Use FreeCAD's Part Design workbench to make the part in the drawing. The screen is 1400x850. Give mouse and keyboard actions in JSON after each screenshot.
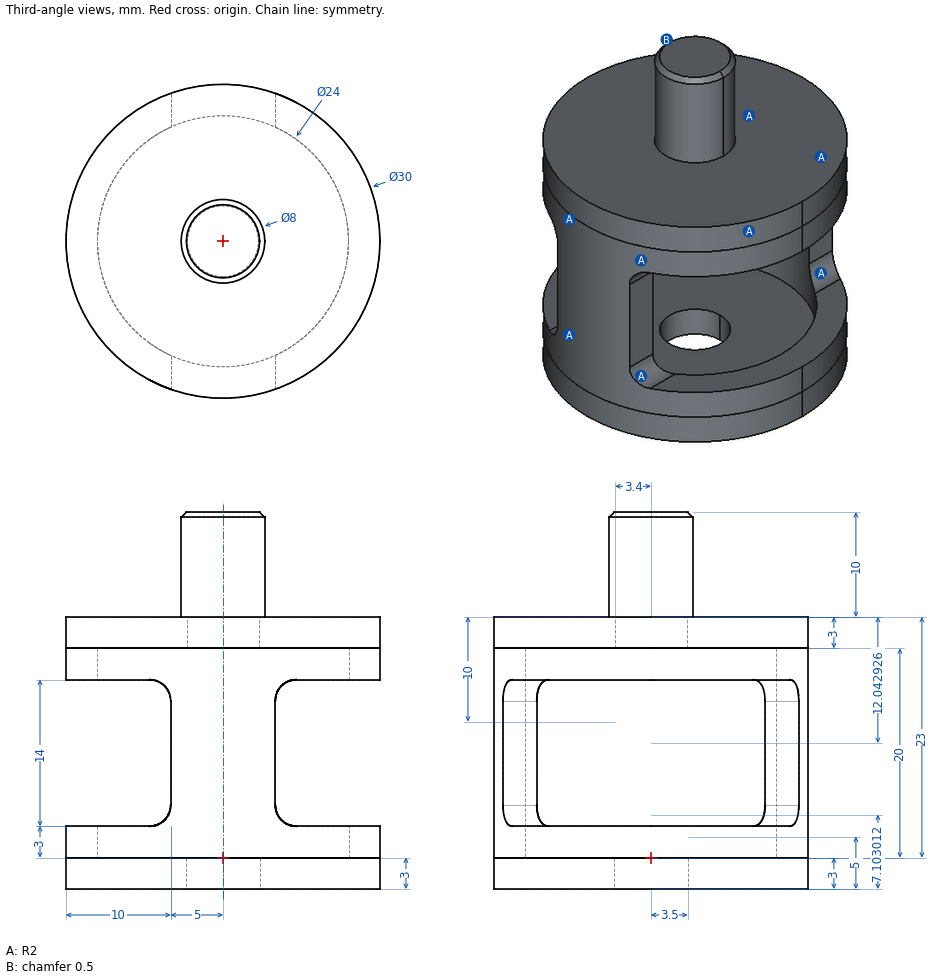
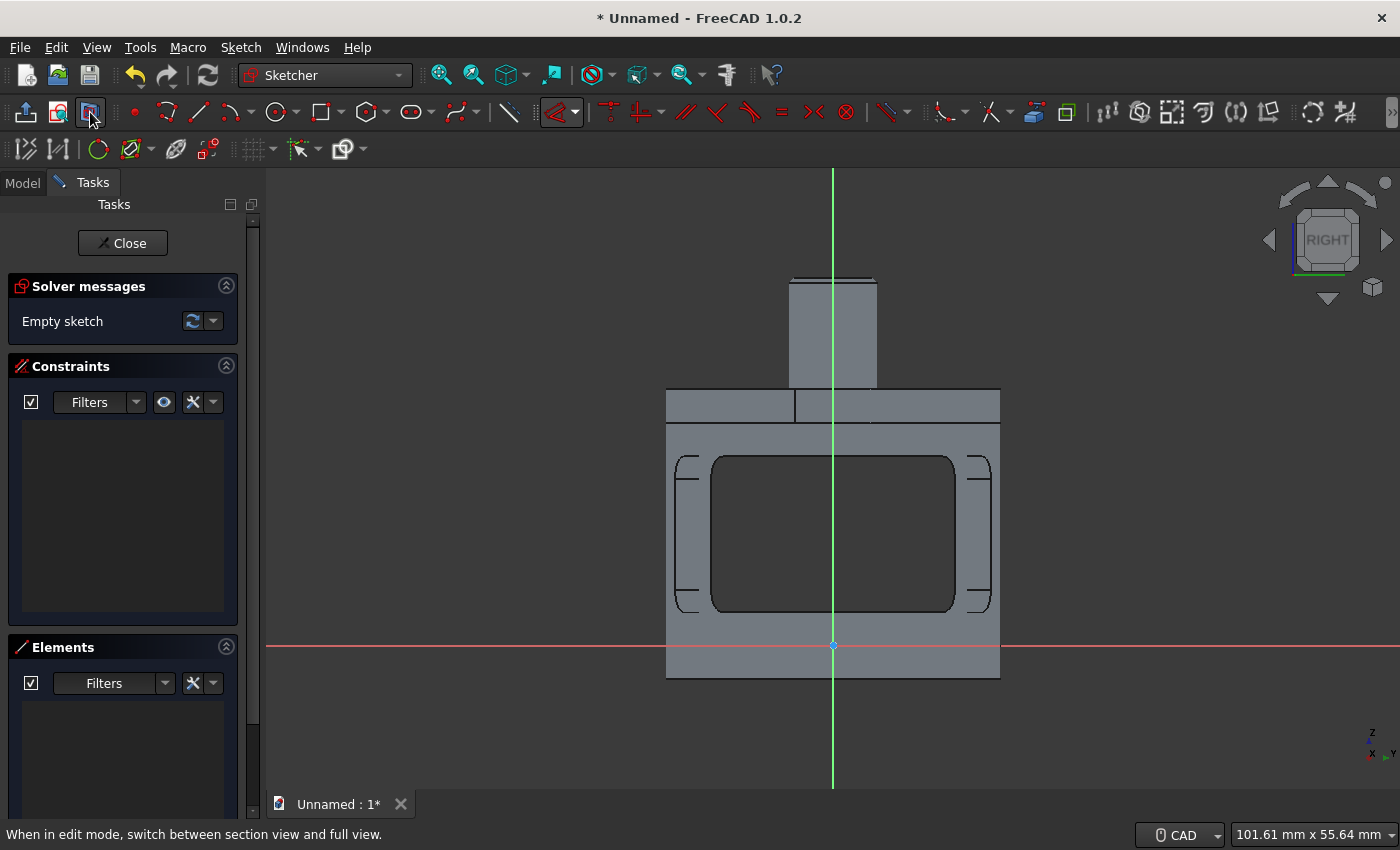
{"action": "scroll", "coordinate": [875, 681], "scroll_direction": "up", "scroll_amount": 8}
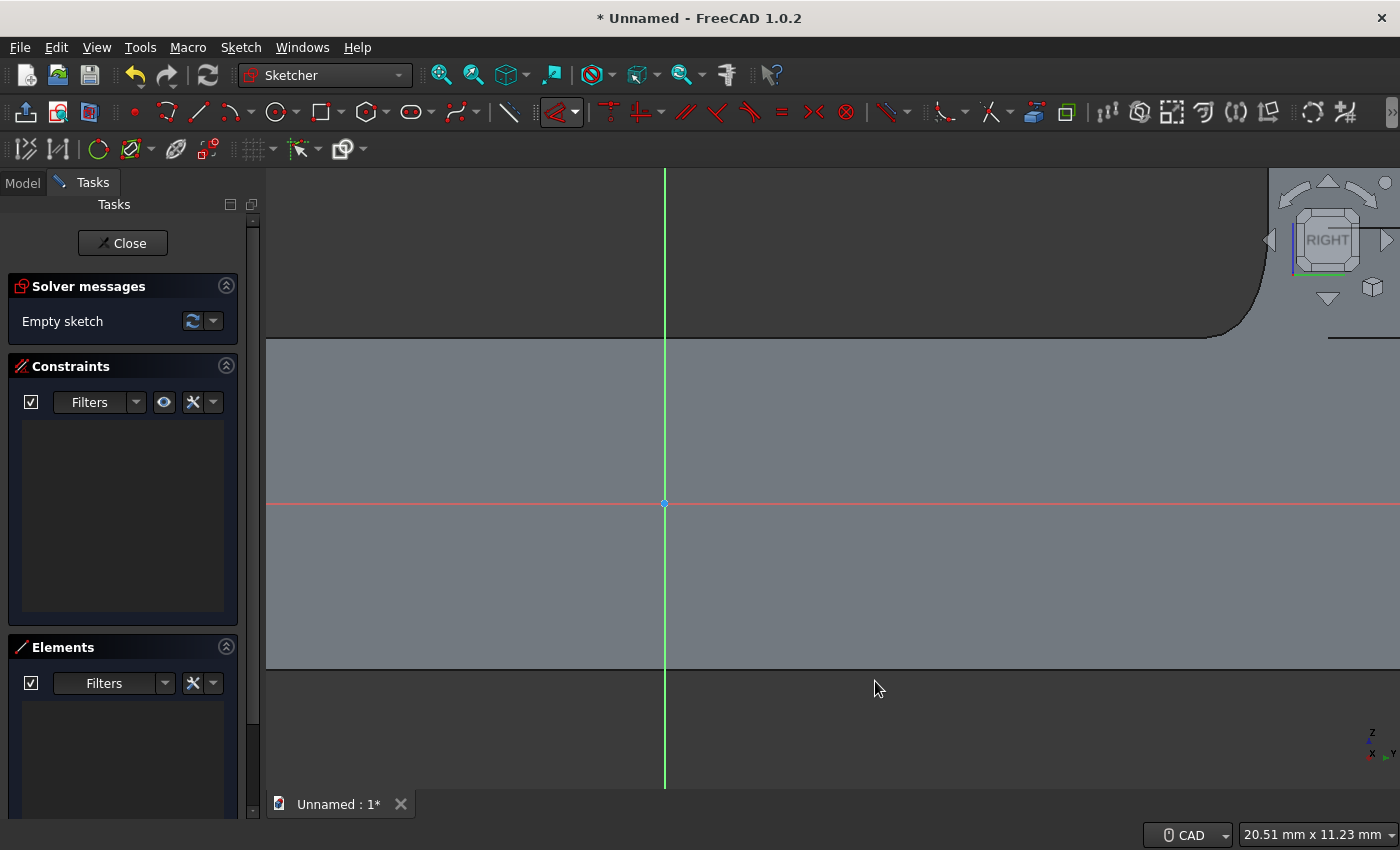
{"action": "key", "text": "g m"}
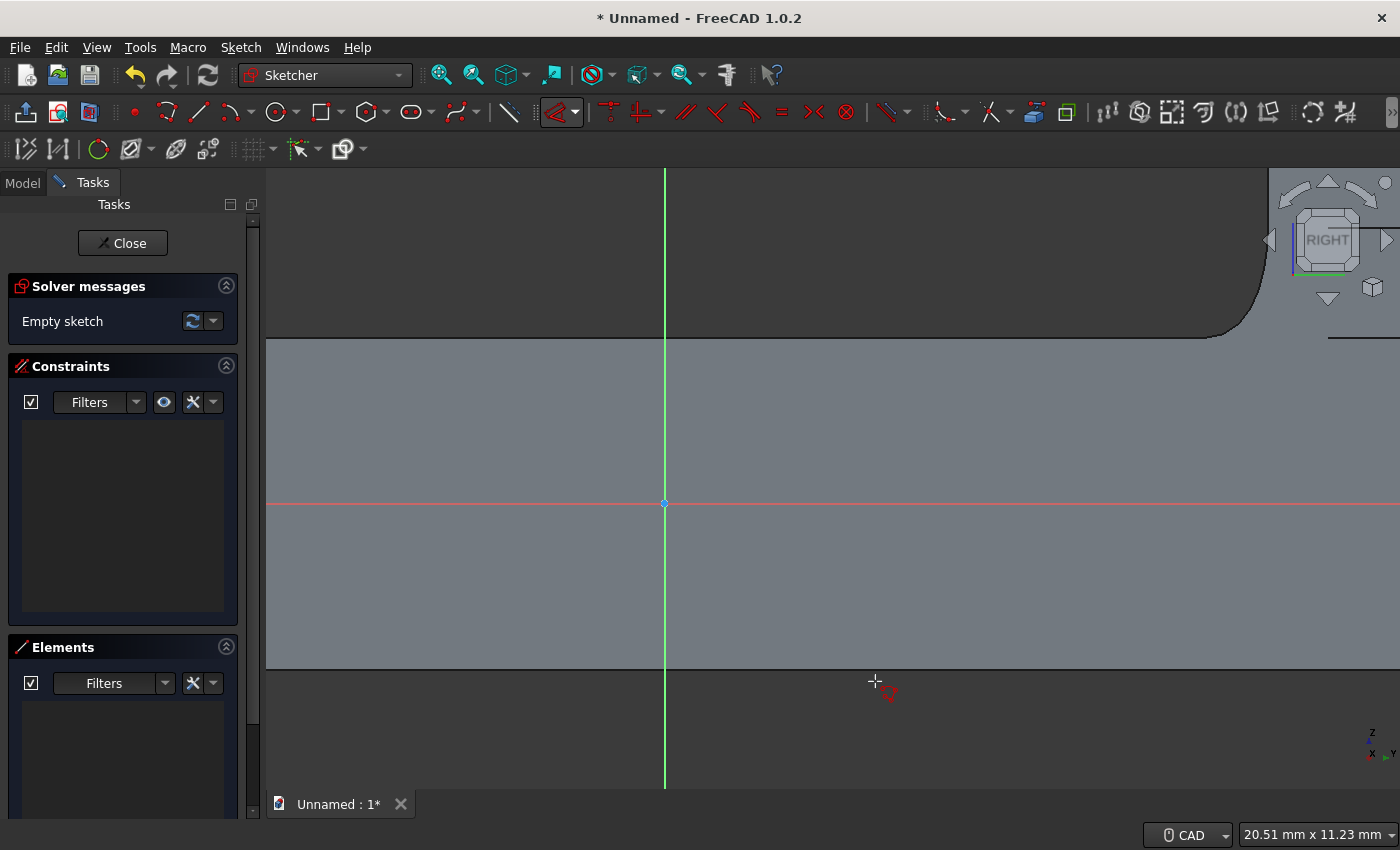
{"action": "left_click", "coordinate": [665, 670]}
{"action": "left_click", "coordinate": [858, 670]}
{"action": "left_click", "coordinate": [858, 393]}
{"action": "left_click", "coordinate": [674, 277]}
{"action": "left_click", "coordinate": [665, 671]}
{"action": "key", "text": "Escape"}
{"action": "key", "text": "Escape"}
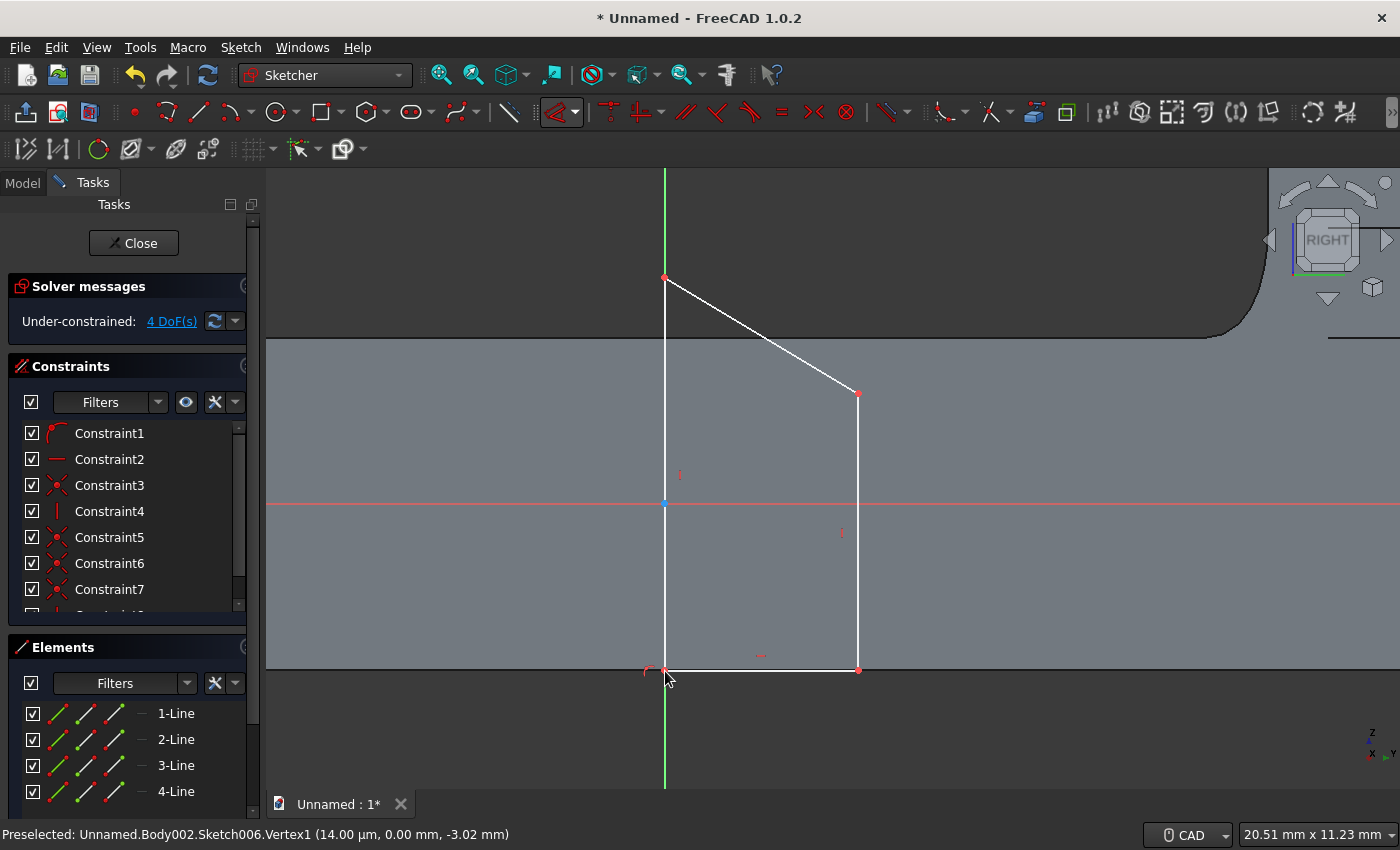
{"action": "left_click", "coordinate": [858, 588]}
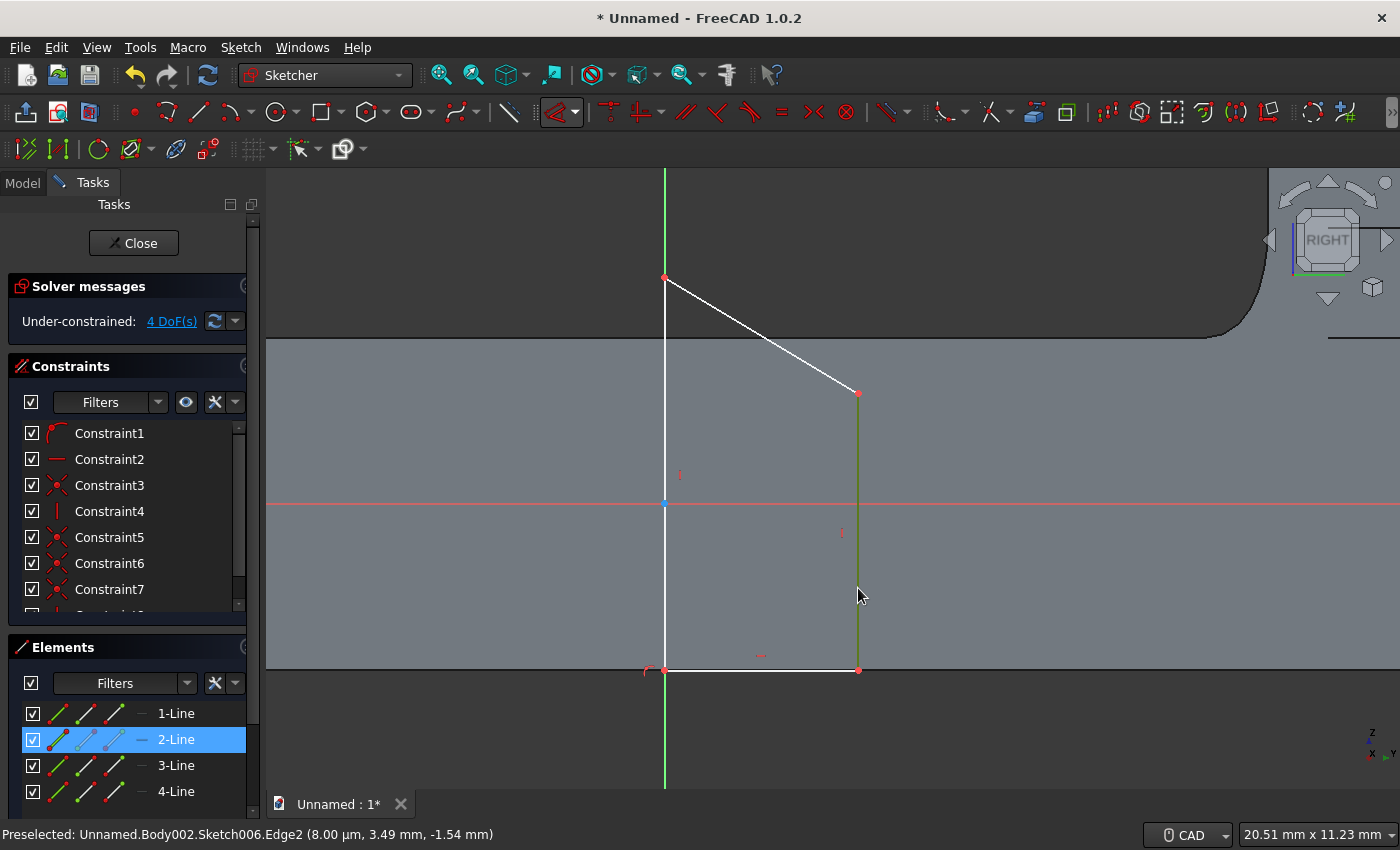
{"action": "key", "text": "i"}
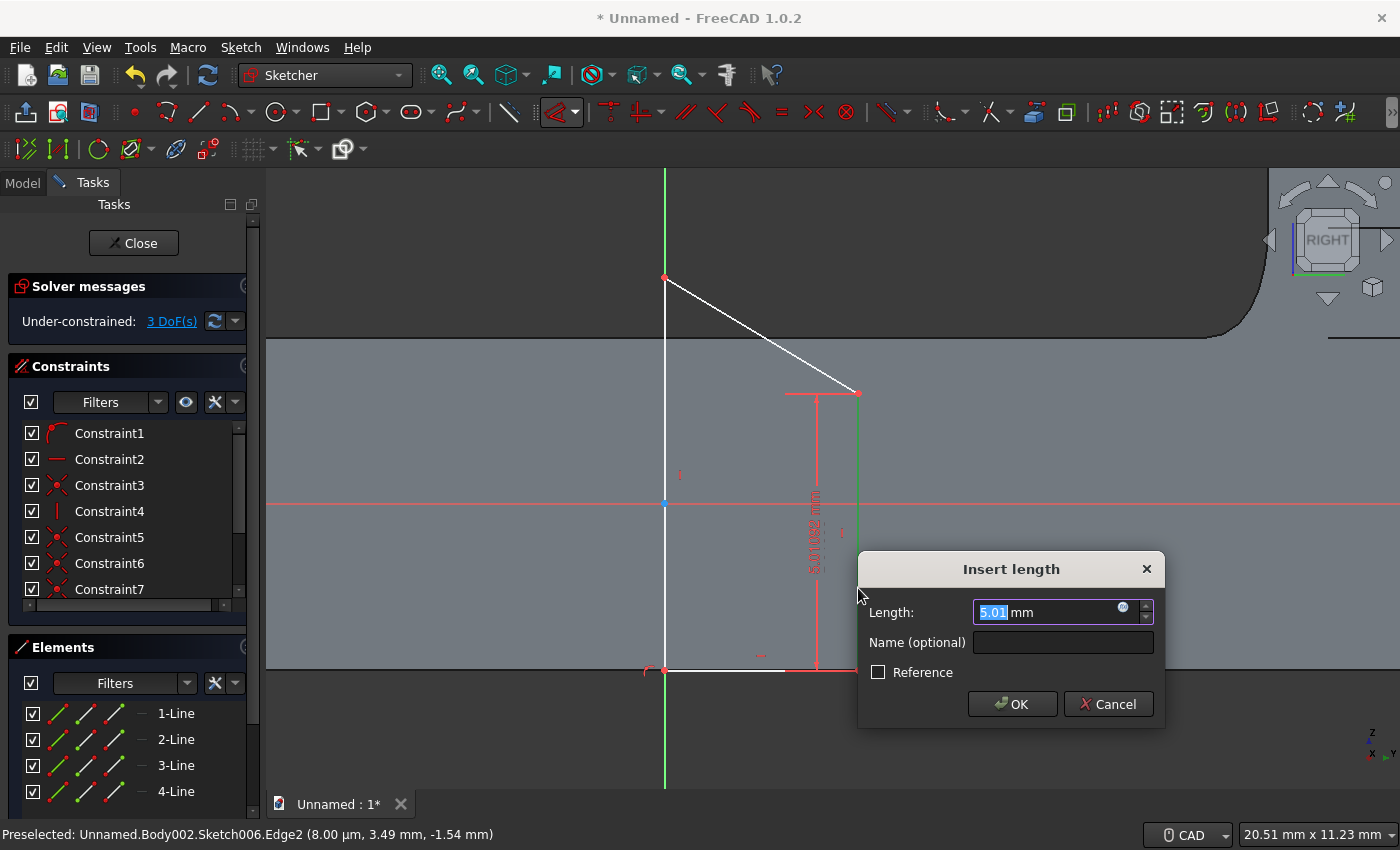
{"action": "type", "text": "5"}
{"action": "key", "text": "Return"}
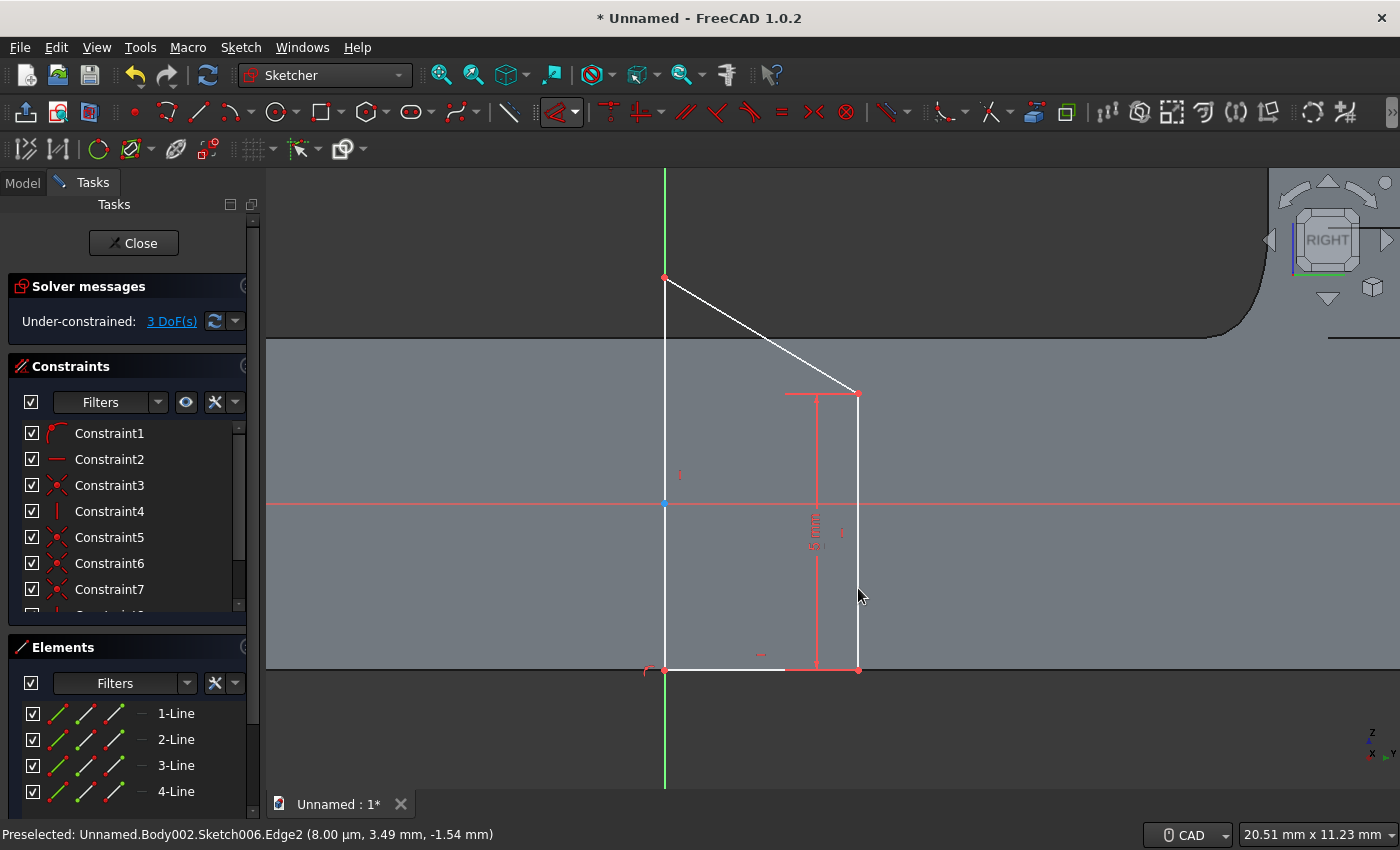
{"action": "left_click", "coordinate": [665, 670]}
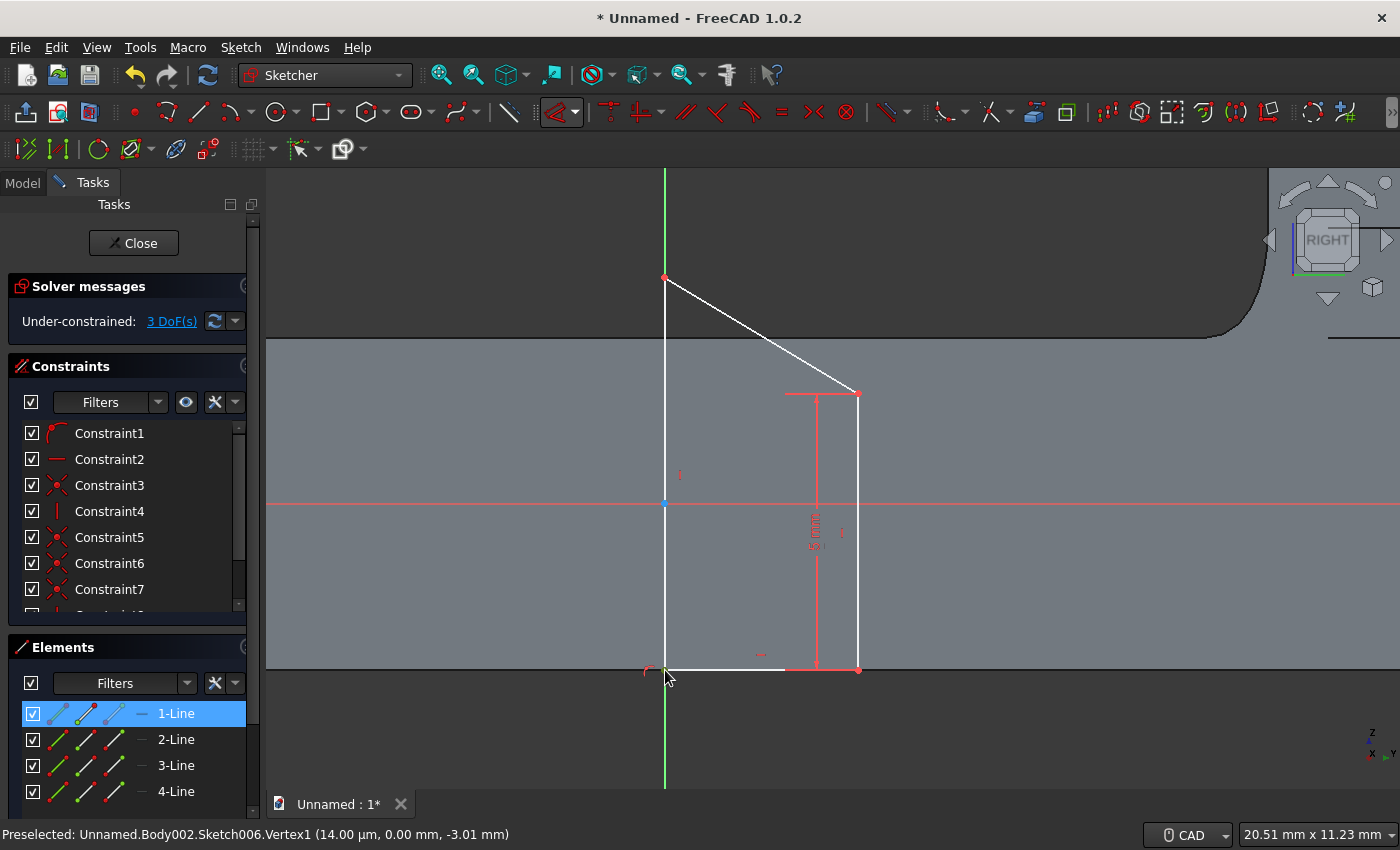
{"action": "left_click", "coordinate": [578, 112]}